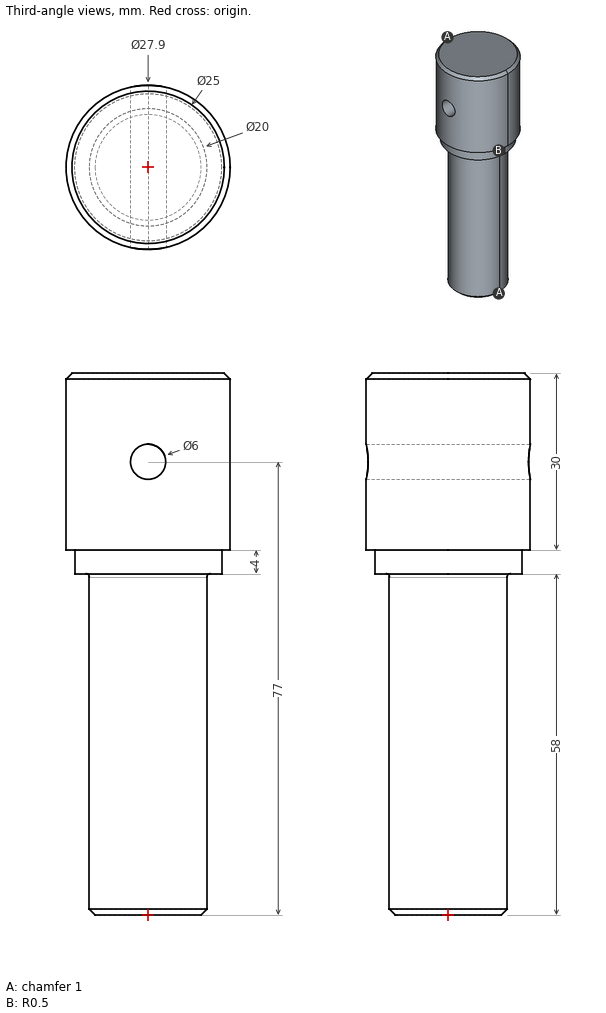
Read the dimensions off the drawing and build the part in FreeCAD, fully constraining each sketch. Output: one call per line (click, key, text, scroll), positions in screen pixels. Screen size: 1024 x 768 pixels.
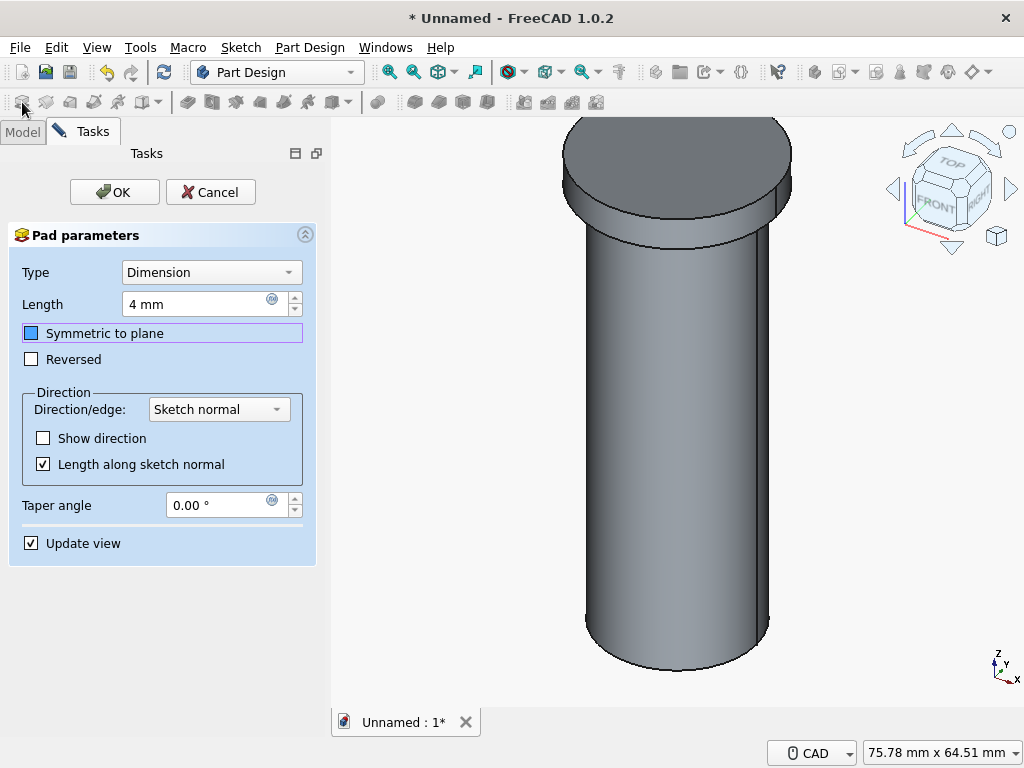
click(115, 192)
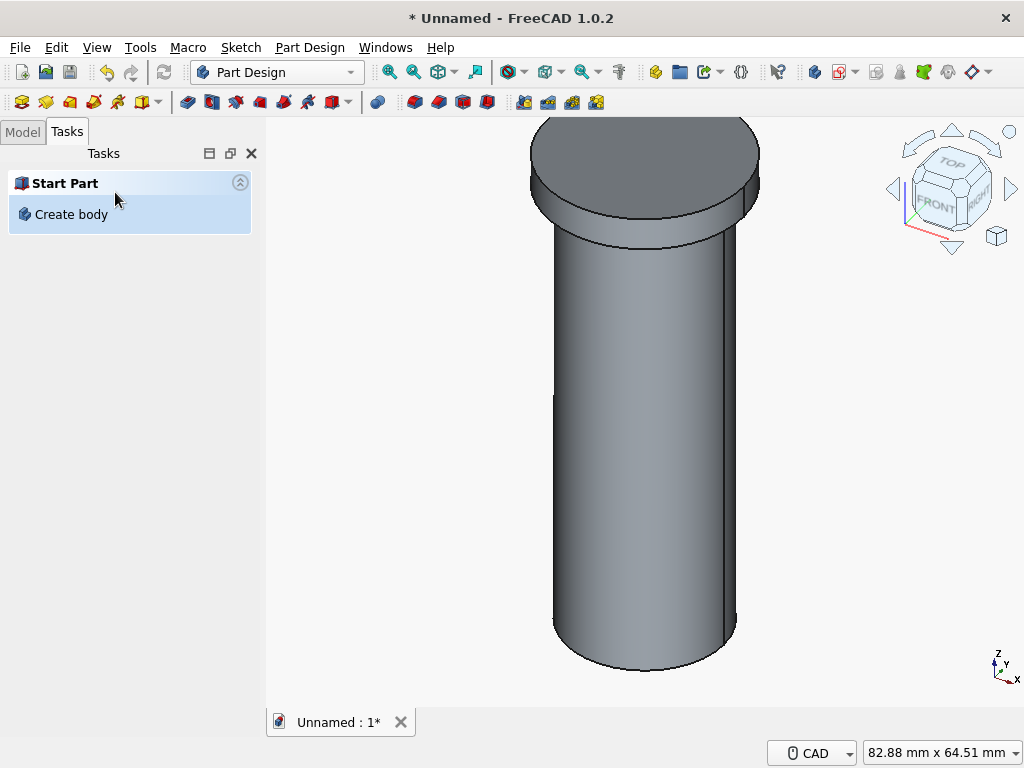
click(390, 72)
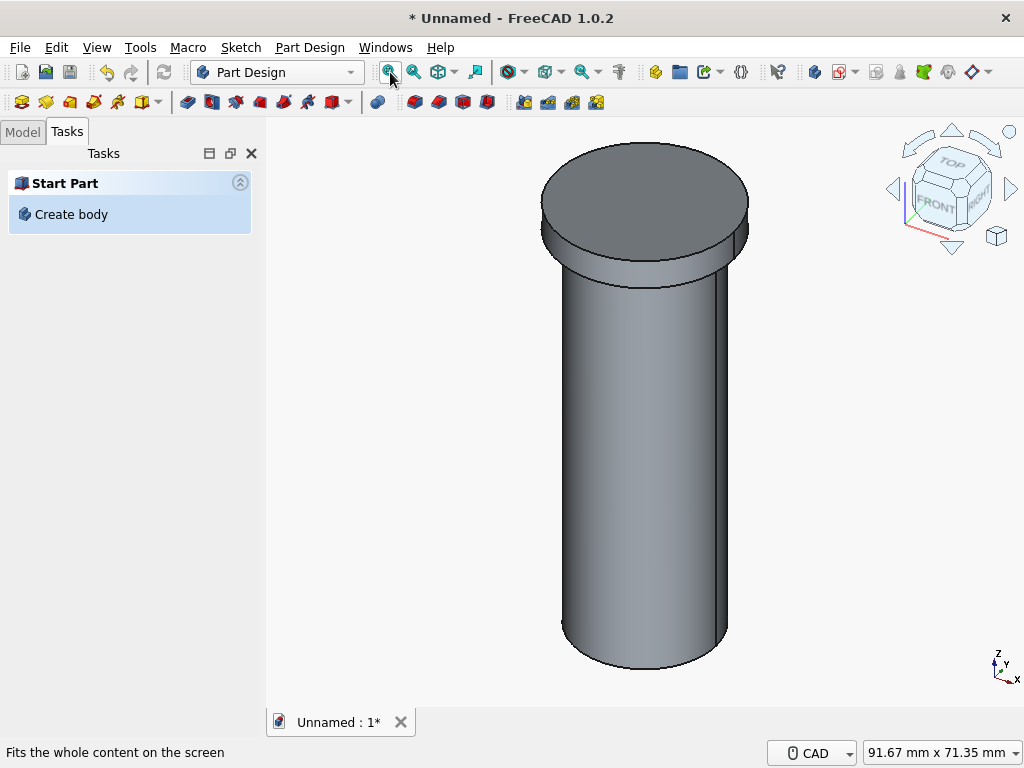
click(645, 201)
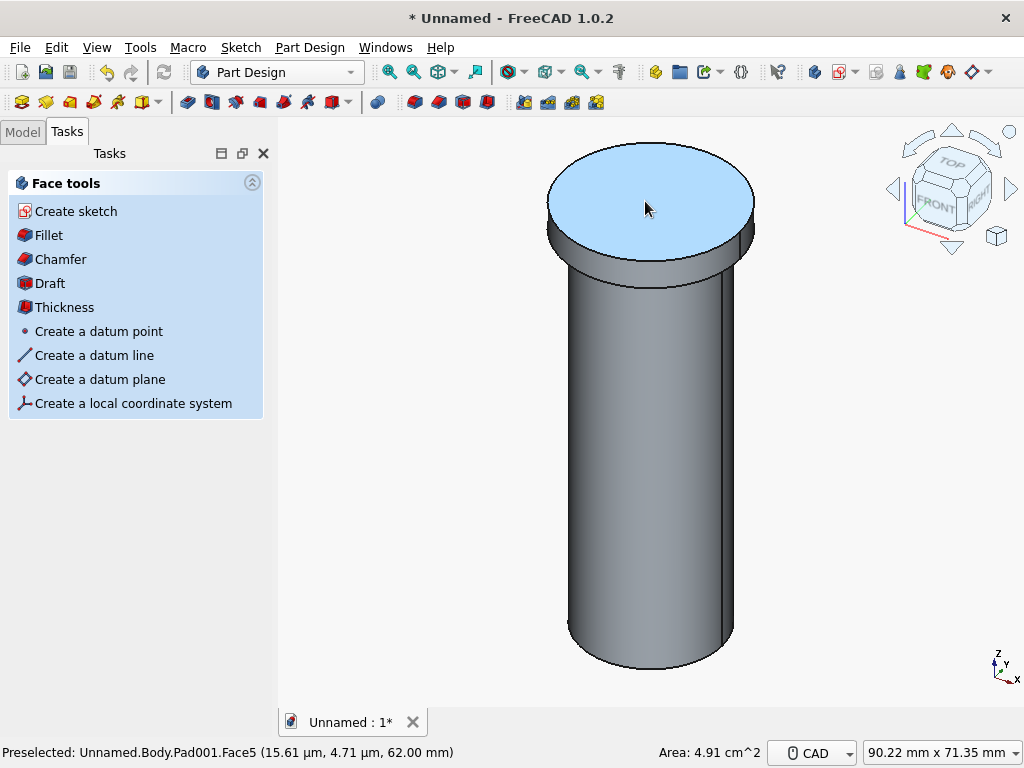
click(840, 72)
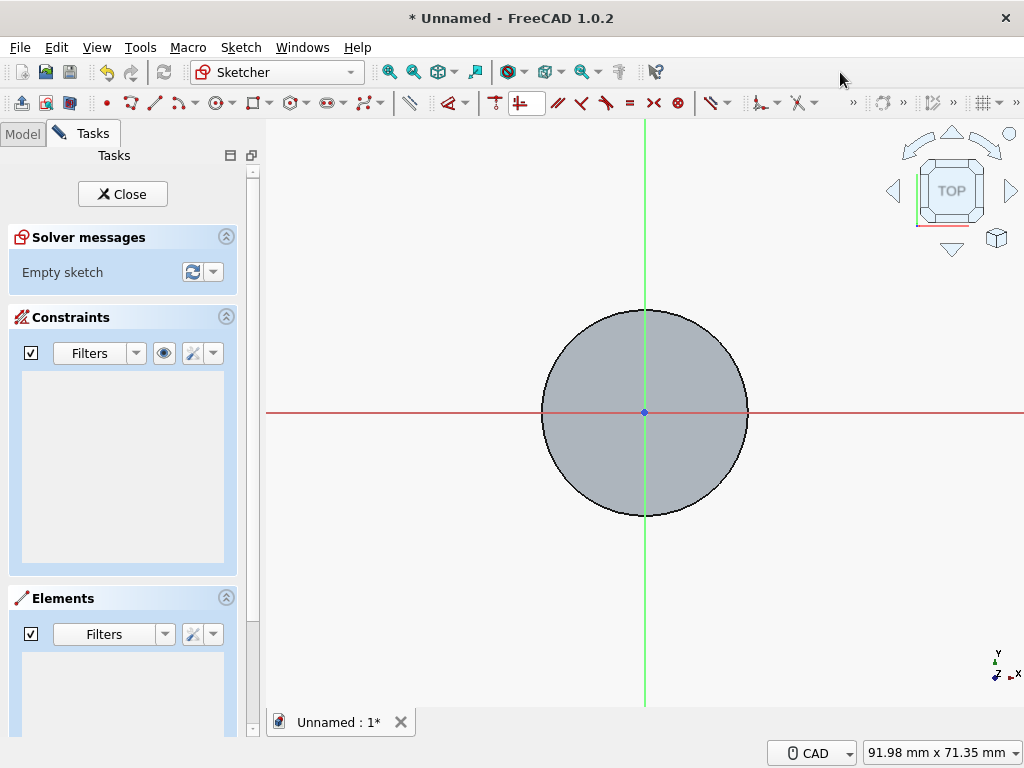
scroll(784, 413, up, 2)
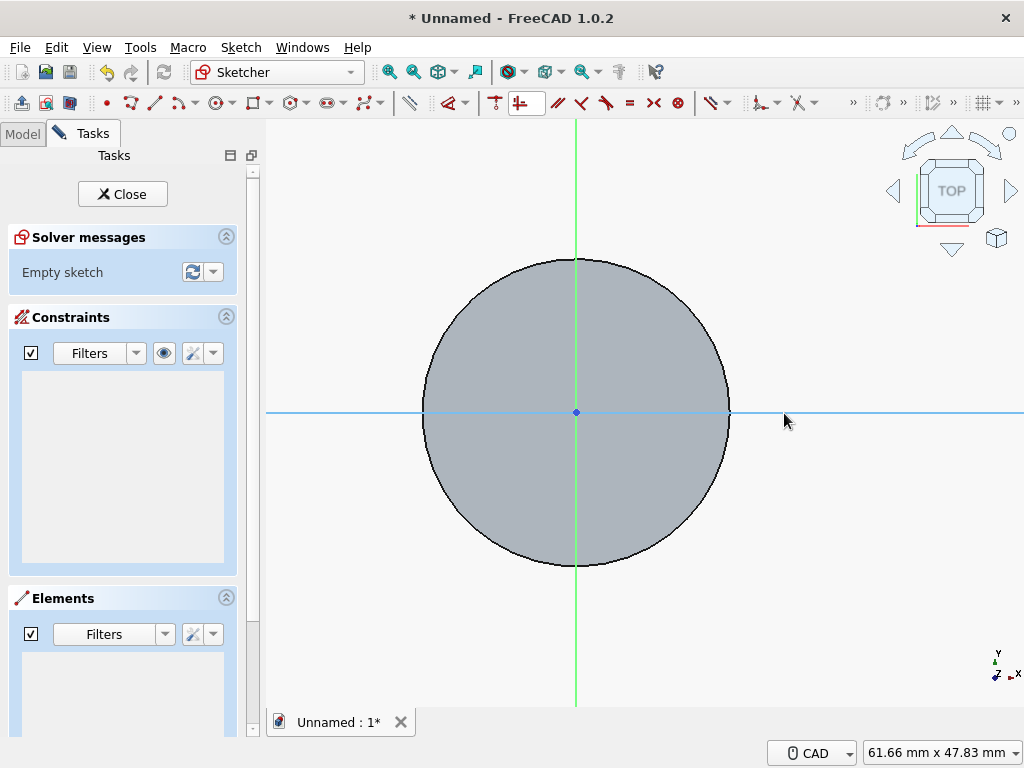
click(216, 104)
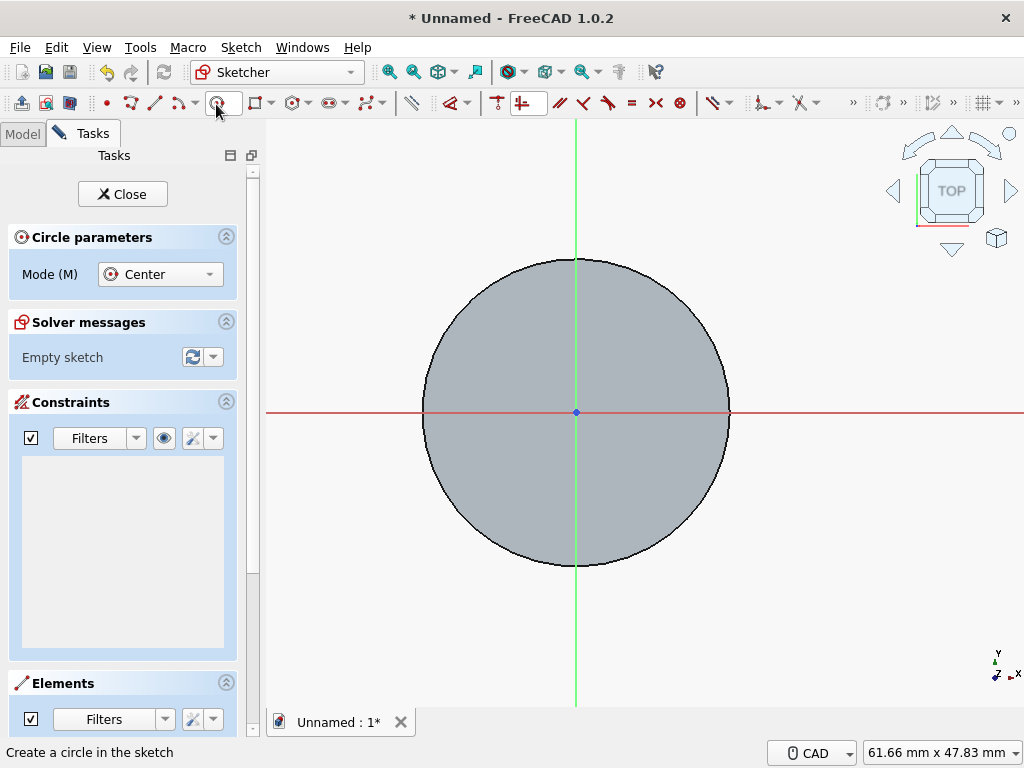
click(576, 413)
click(697, 291)
key(Escape)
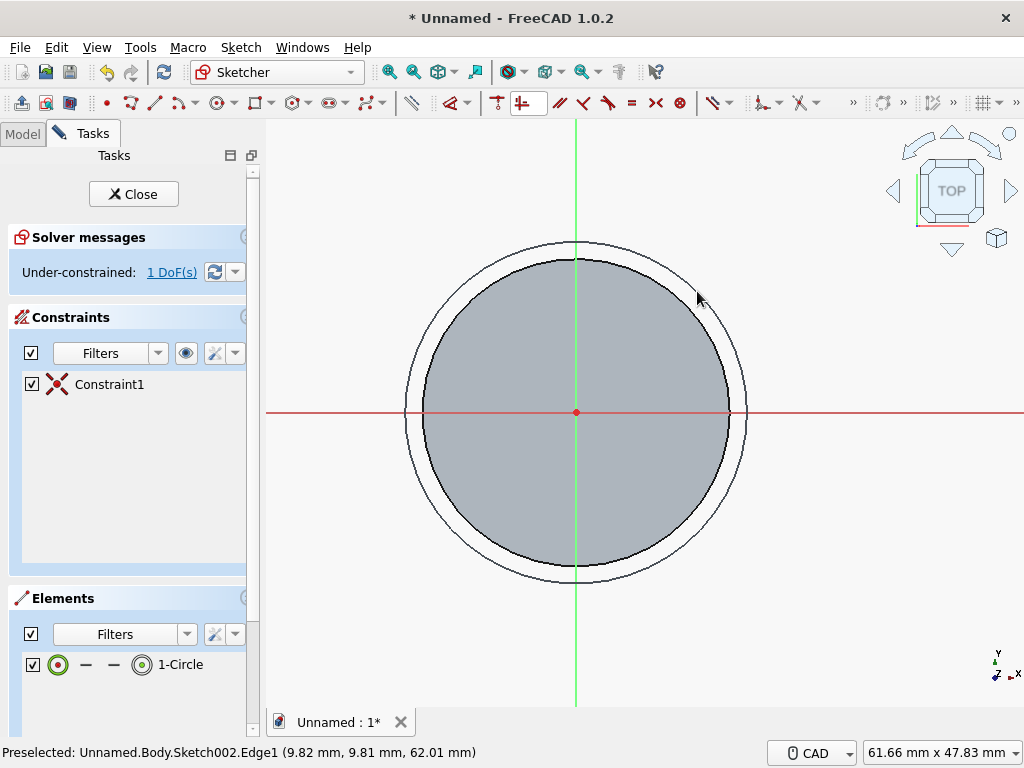
click(450, 104)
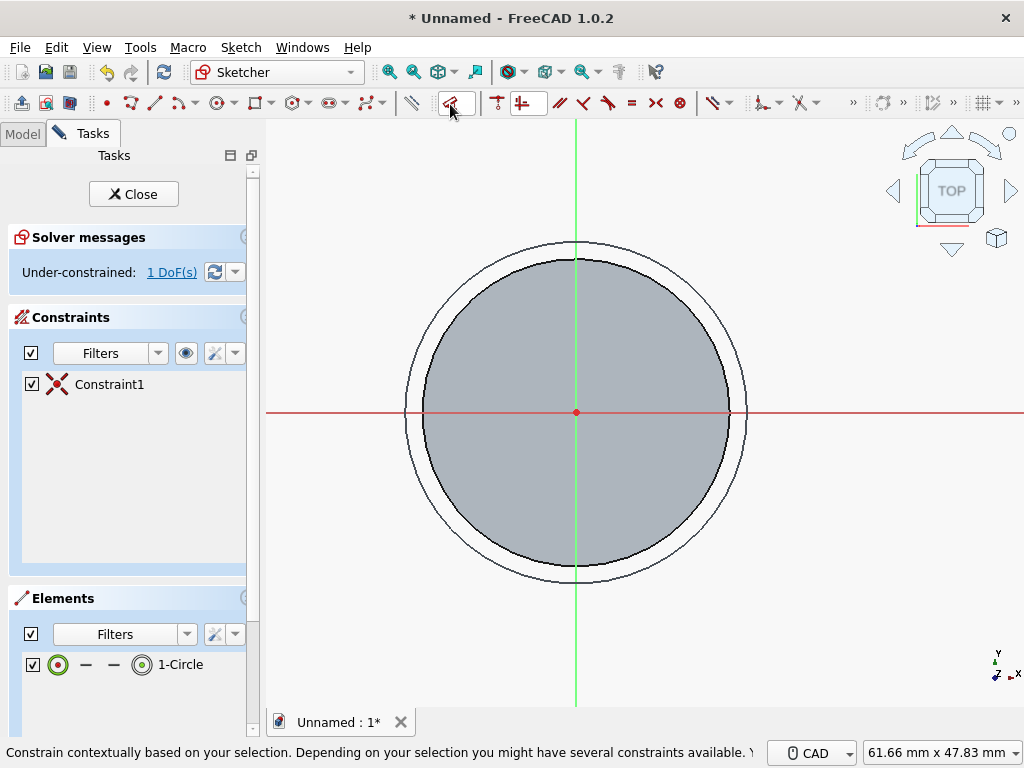
click(697, 292)
click(720, 269)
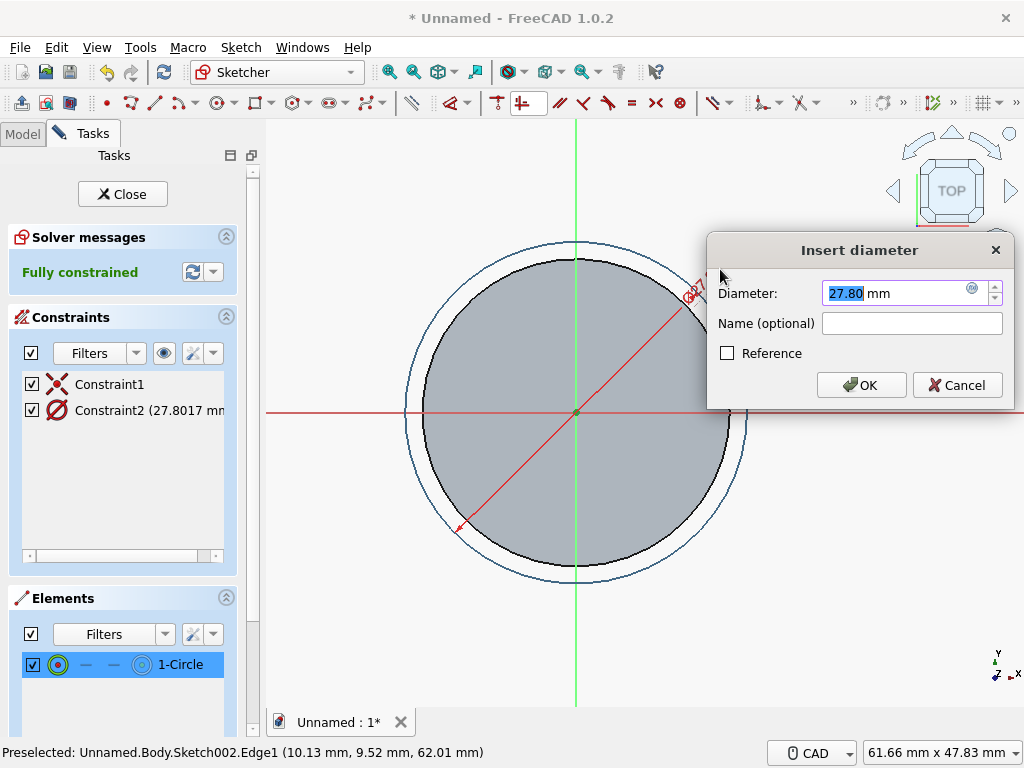
text(27.9)
key(Return)
key(Escape)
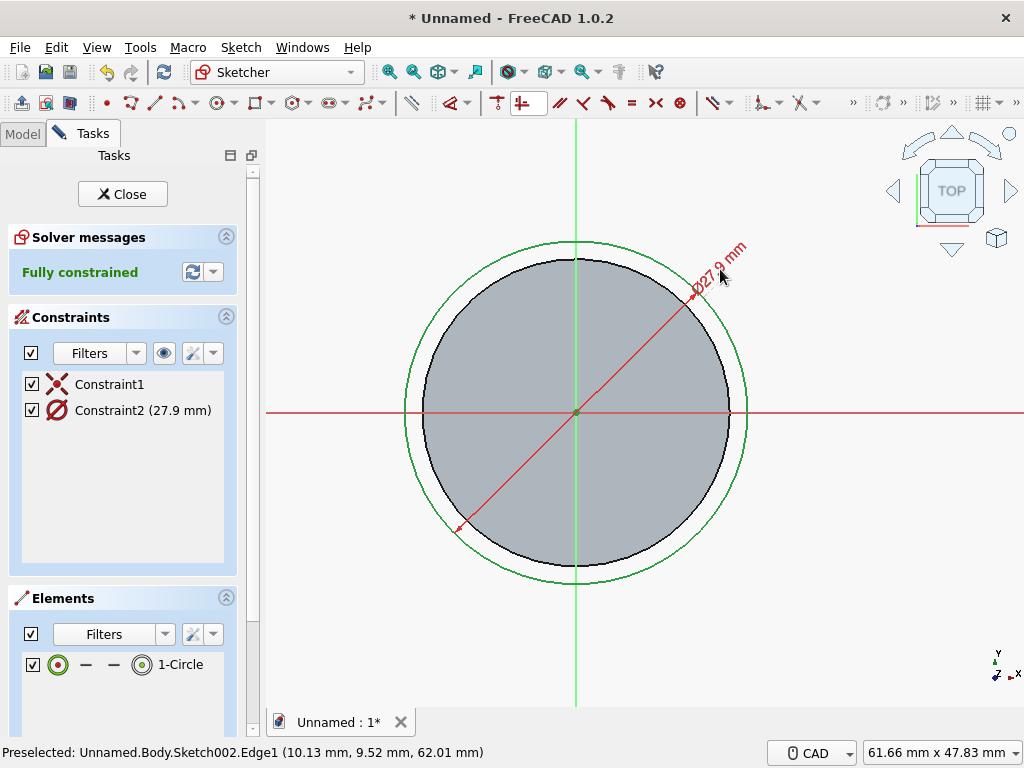
click(123, 194)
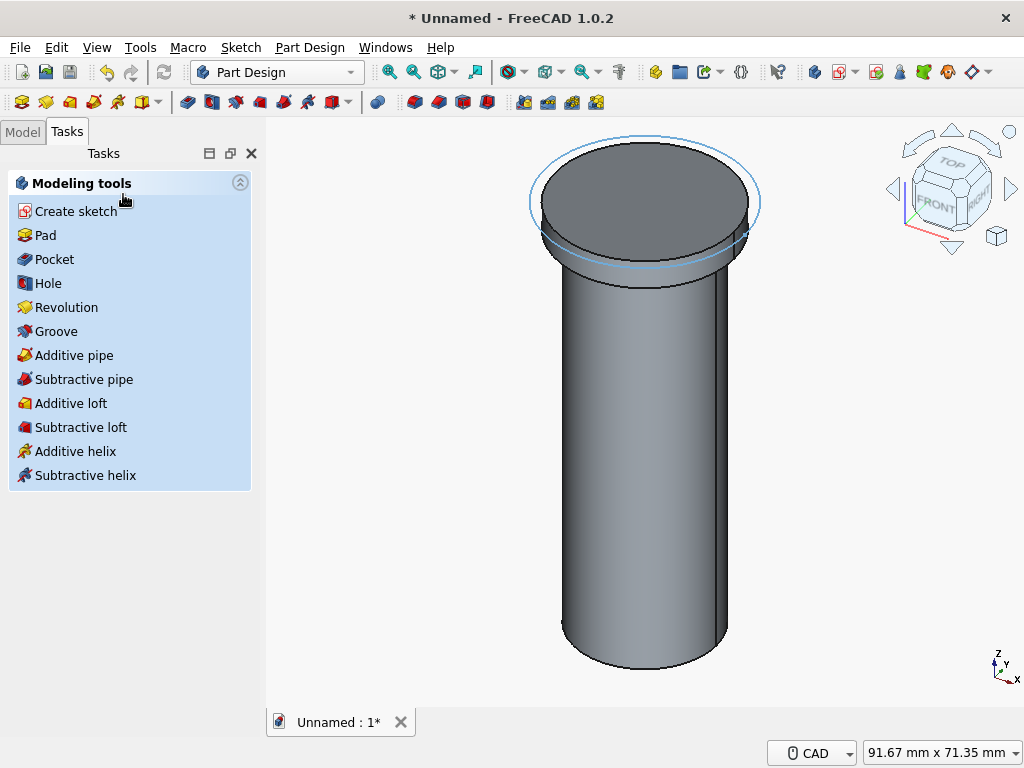
click(22, 102)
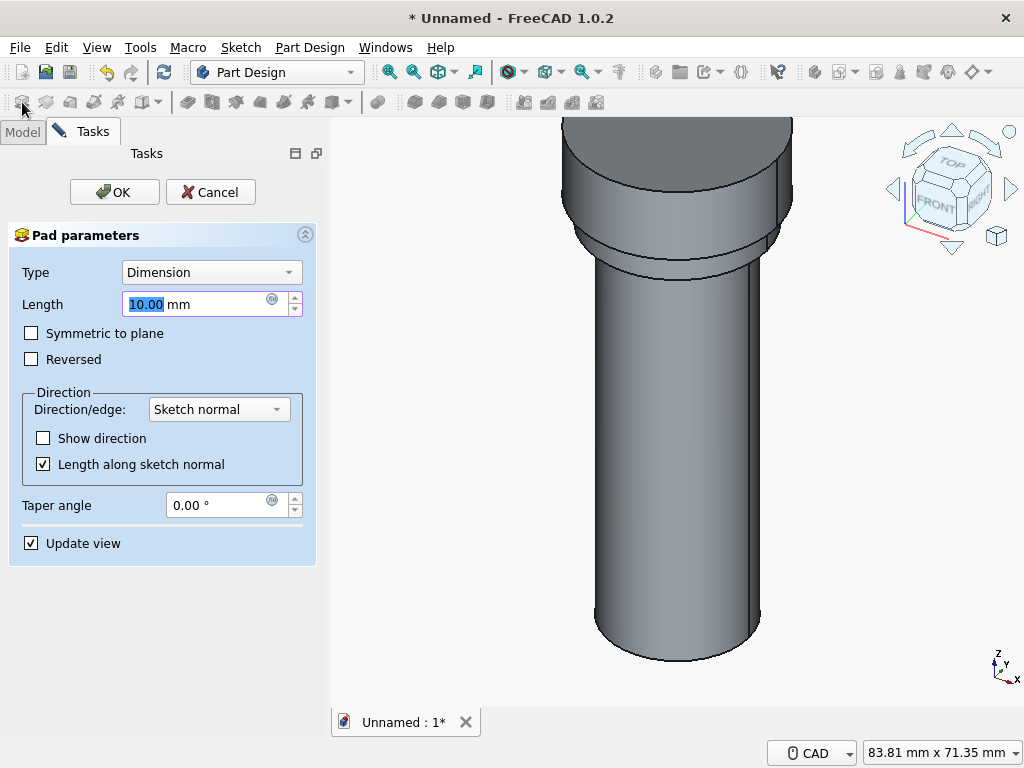
text(30)
key(Tab)